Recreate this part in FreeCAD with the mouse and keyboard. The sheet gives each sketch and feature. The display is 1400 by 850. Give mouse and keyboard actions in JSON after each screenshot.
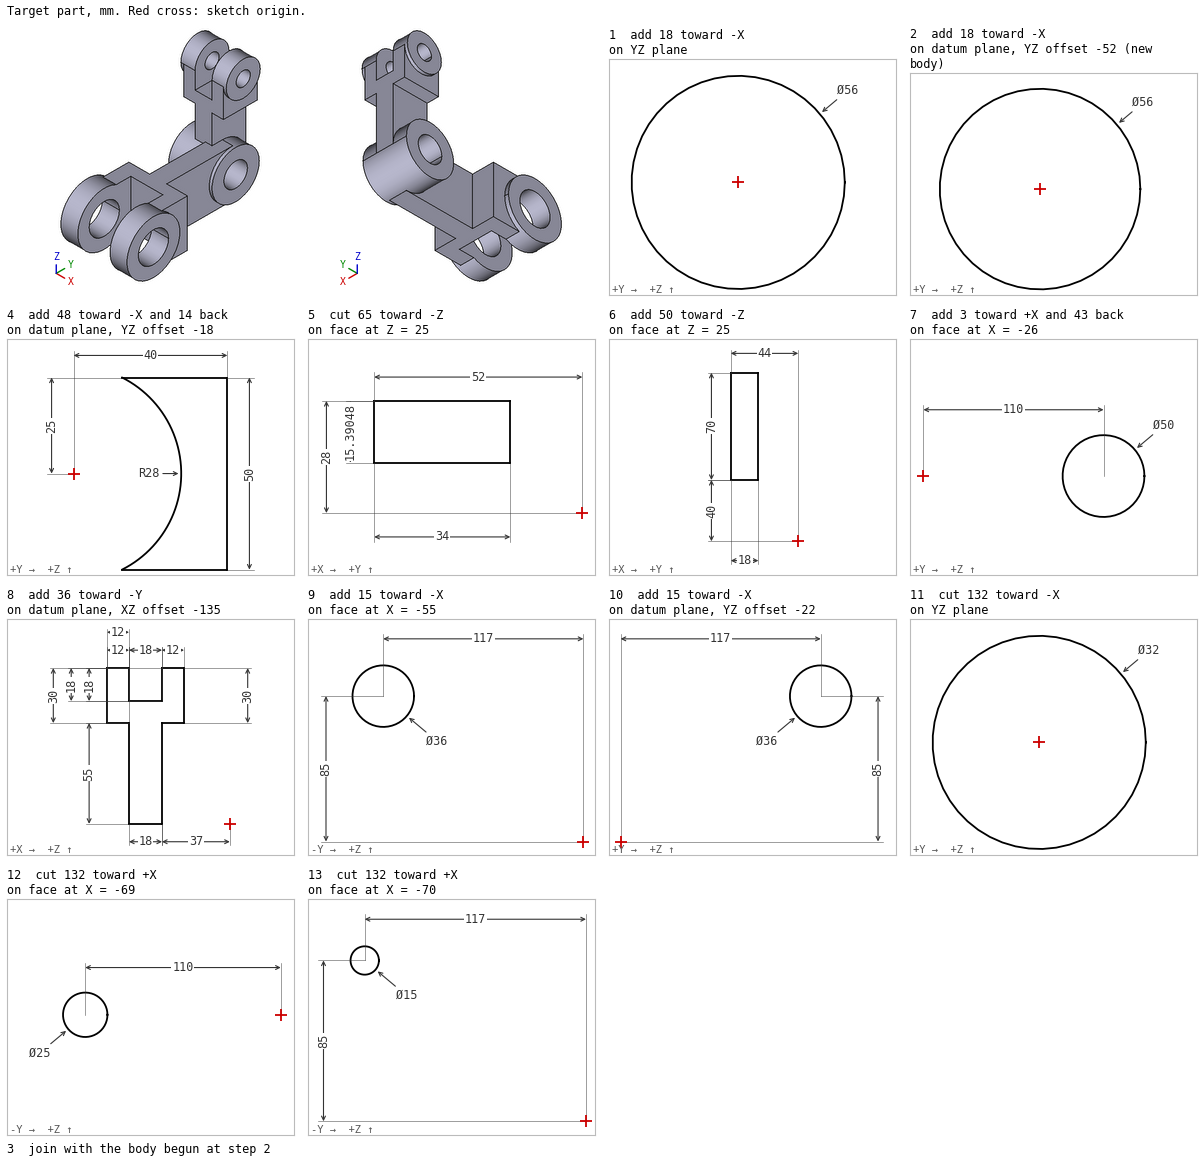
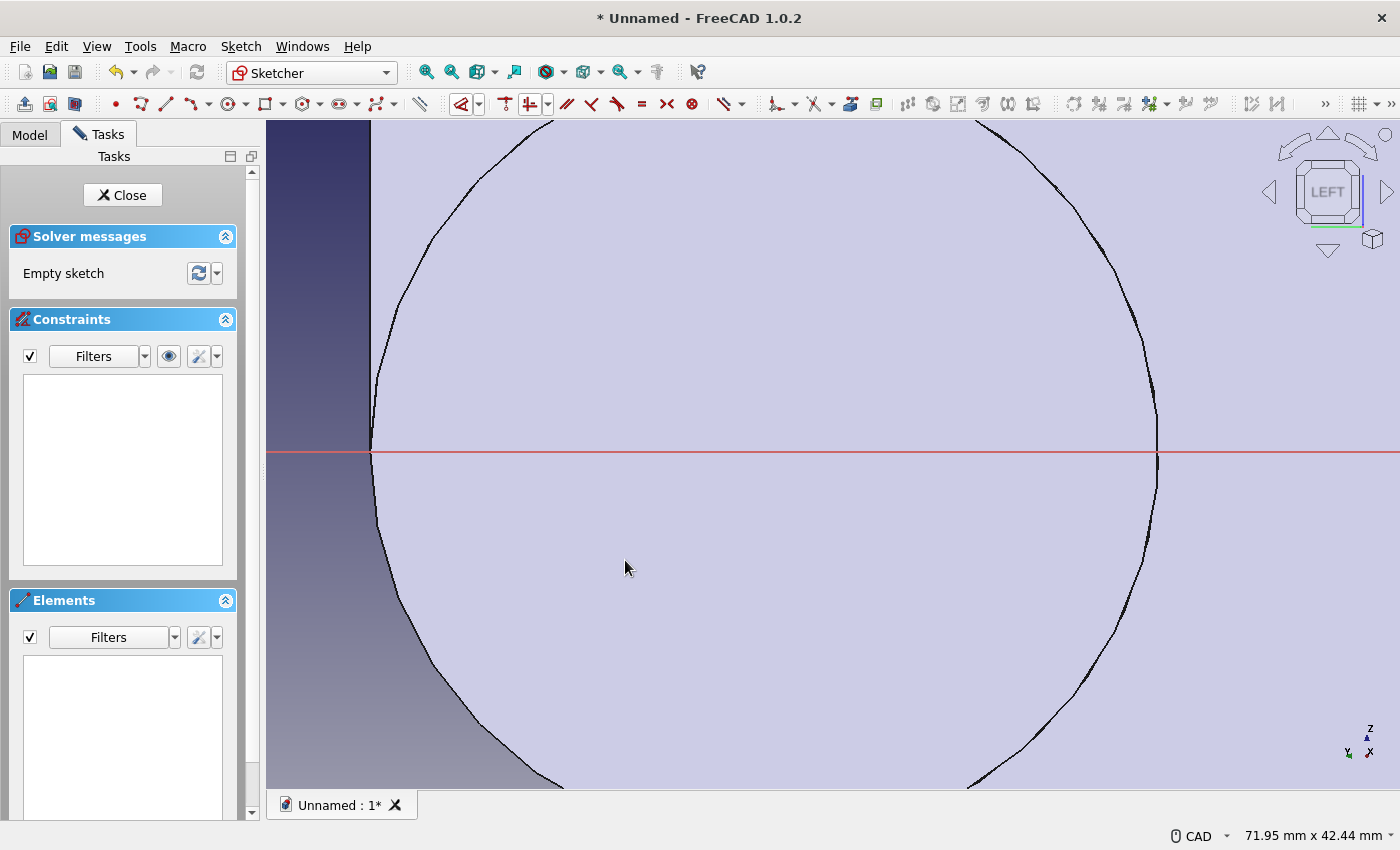
{"action": "left_click", "coordinate": [228, 104]}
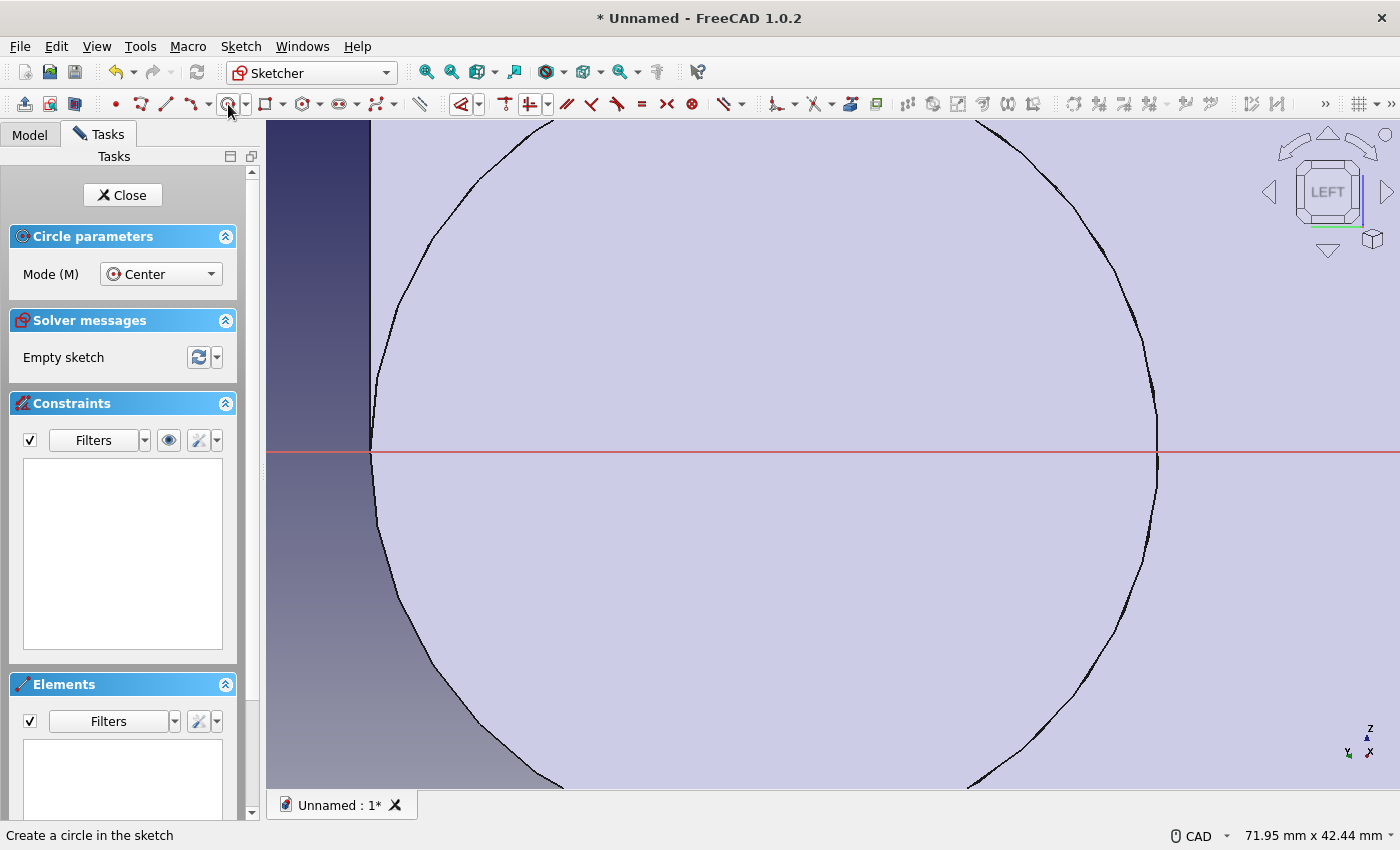
{"action": "left_click", "coordinate": [764, 452]}
{"action": "left_click", "coordinate": [904, 312]}
{"action": "key", "text": "Escape"}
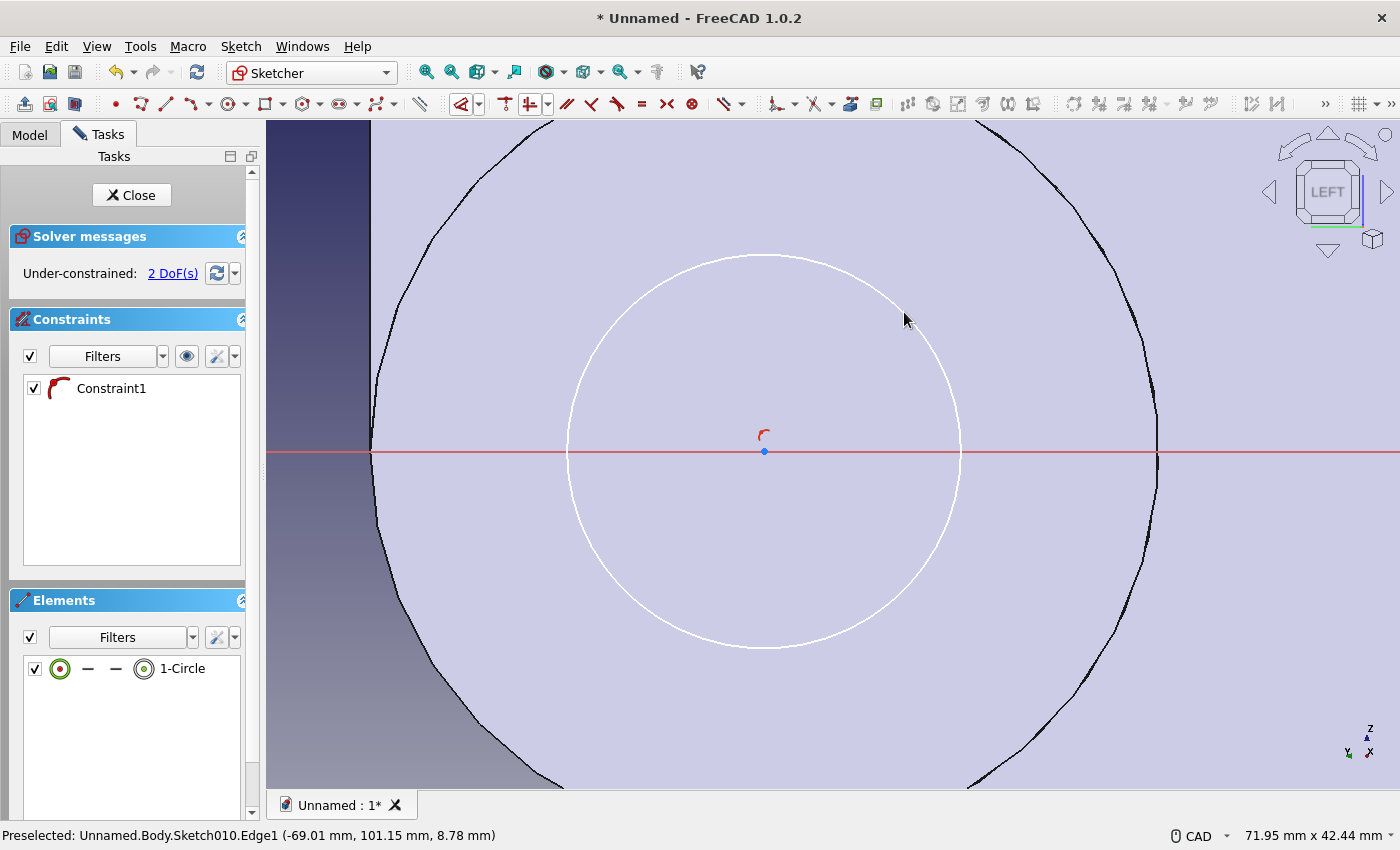
{"action": "left_click", "coordinate": [903, 312]}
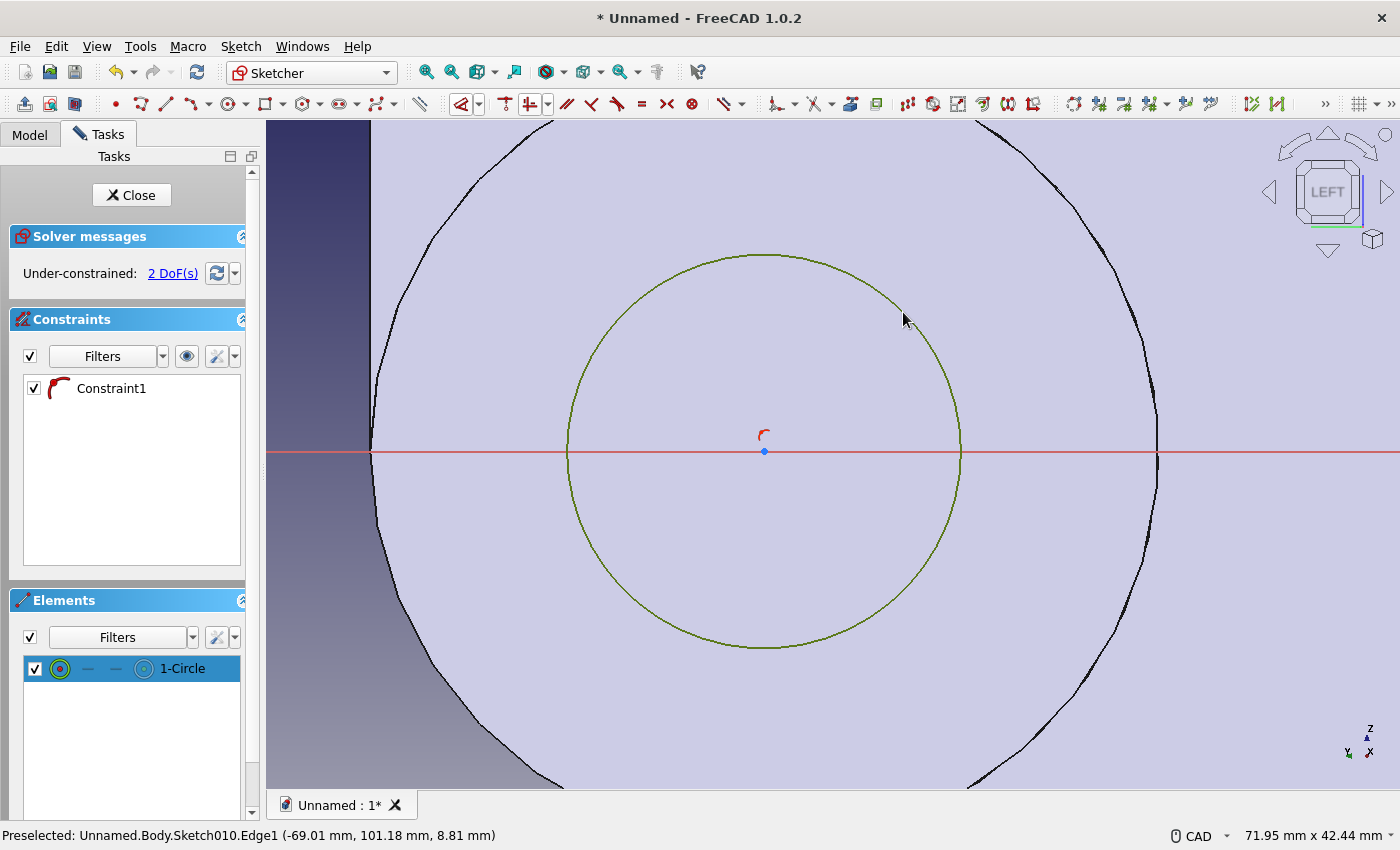
{"action": "key", "text": "k o"}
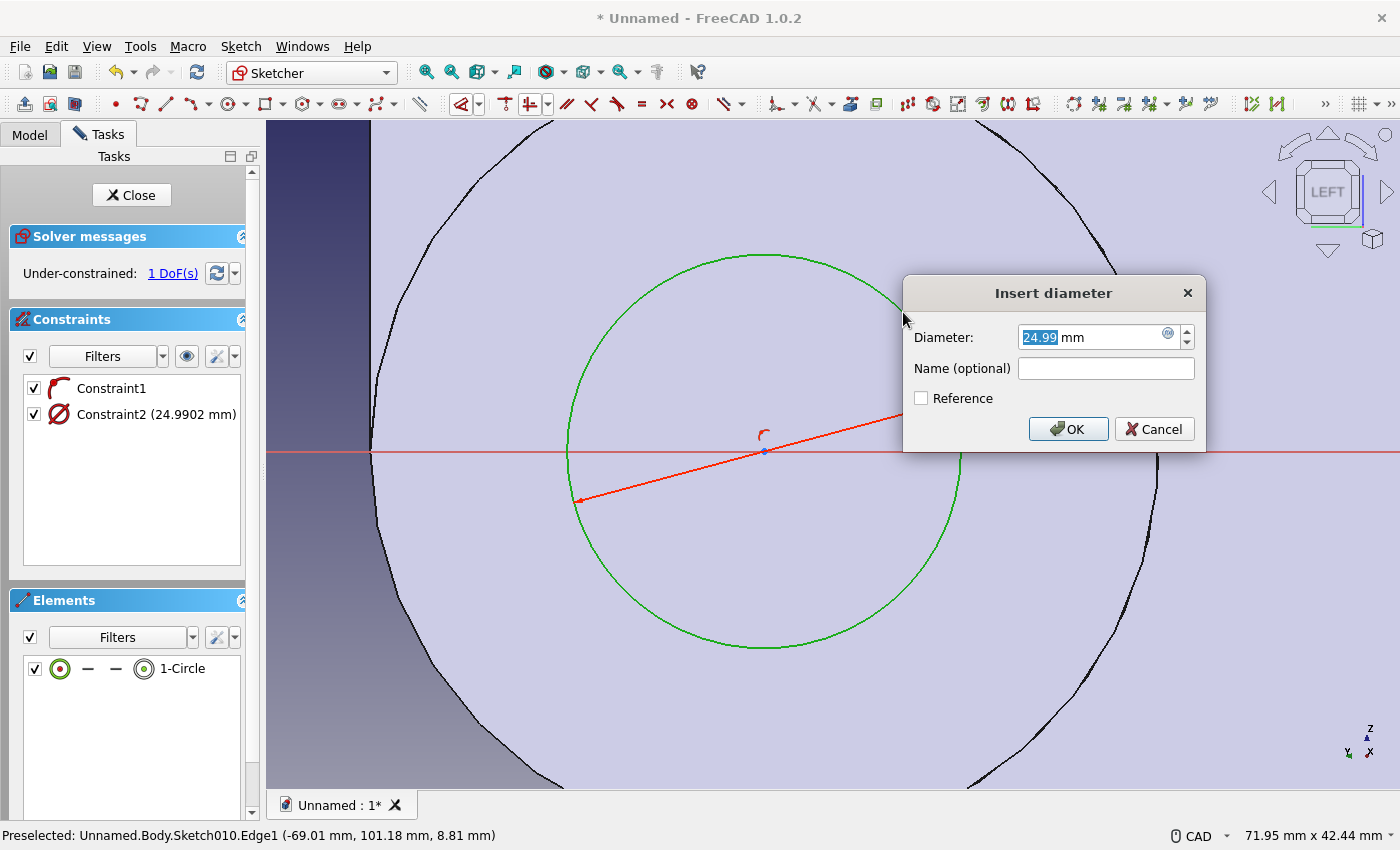
{"action": "type", "text": "25"}
{"action": "key", "text": "Return"}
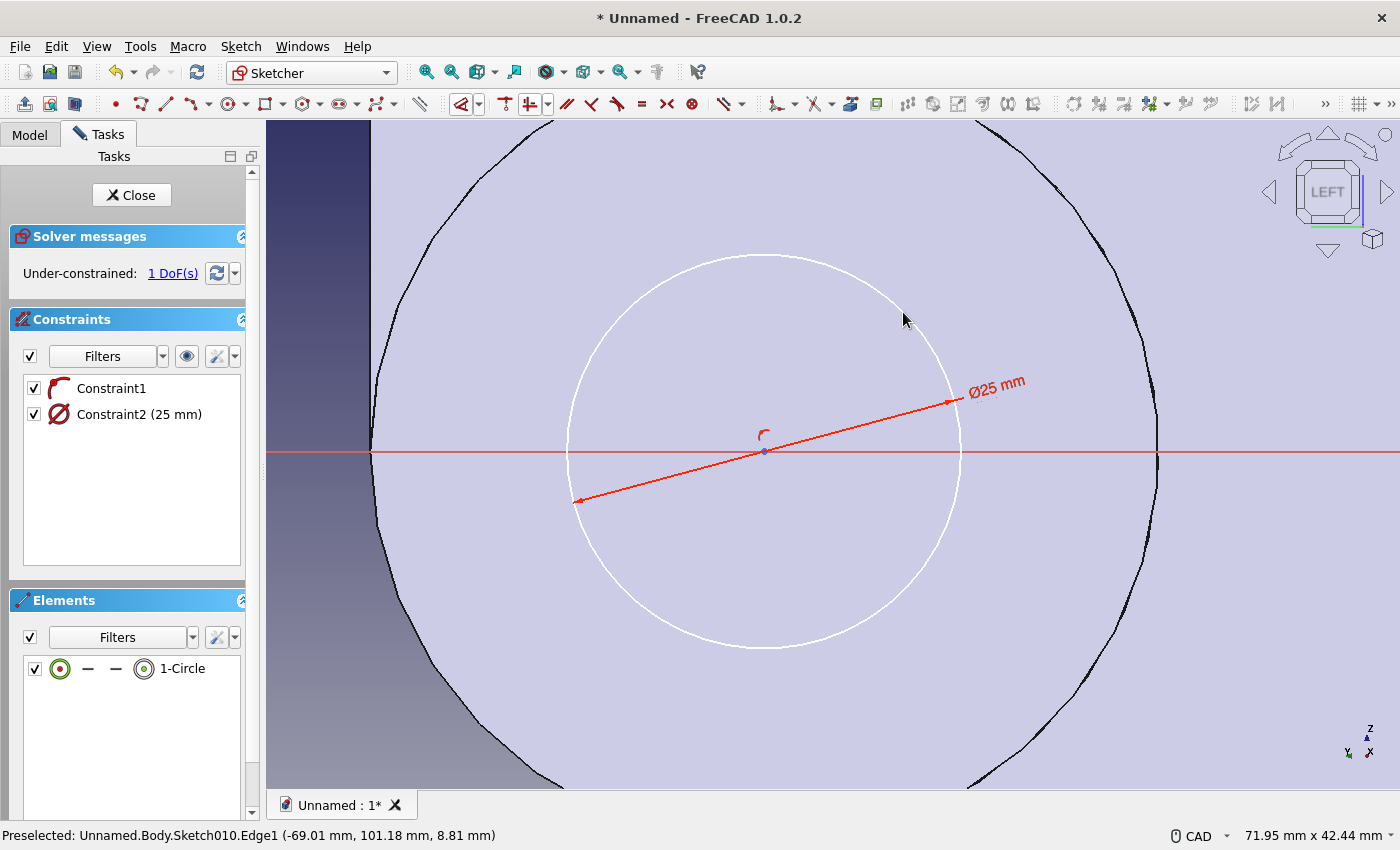
{"action": "left_click", "coordinate": [764, 452]}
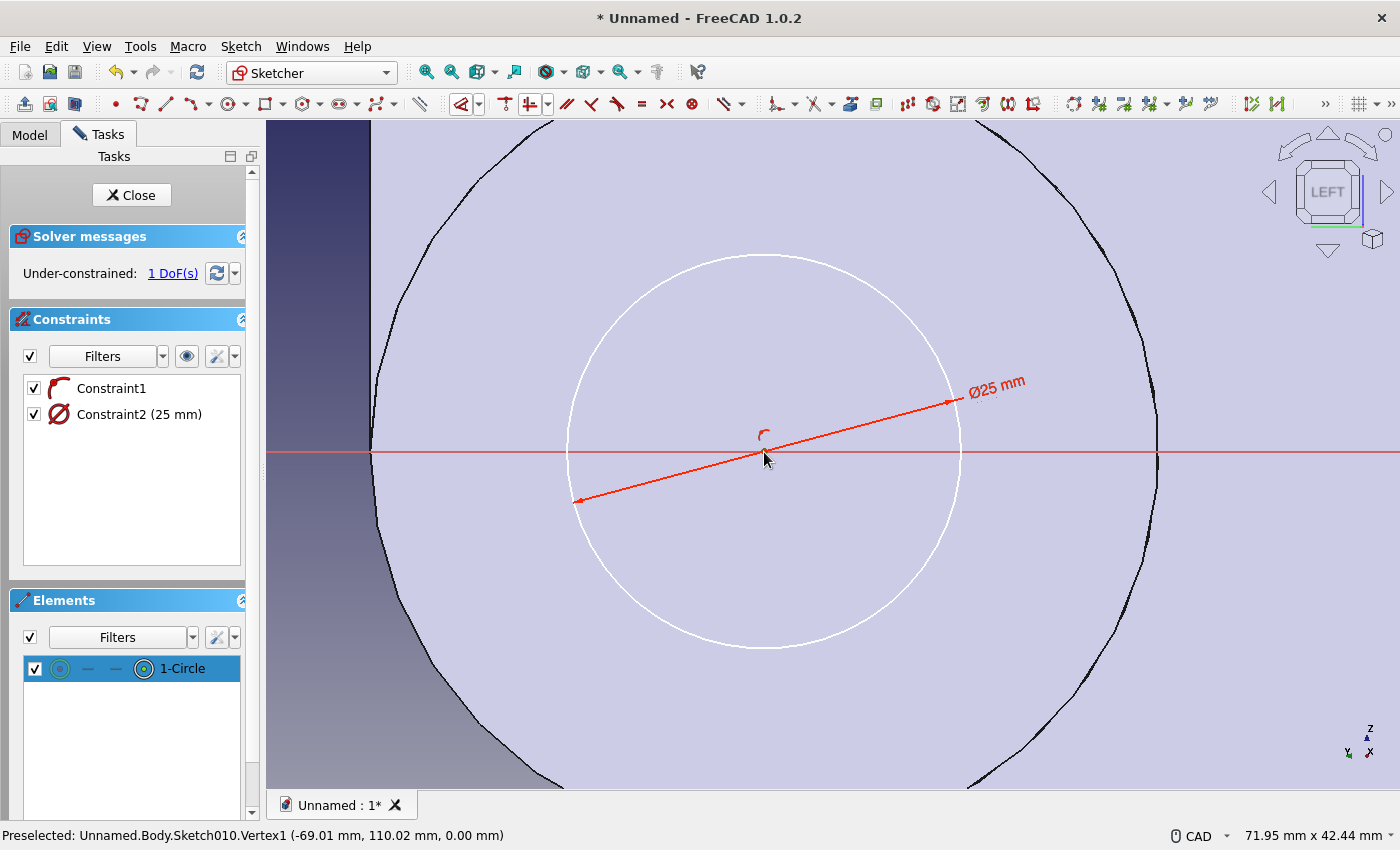
{"action": "key", "text": "l"}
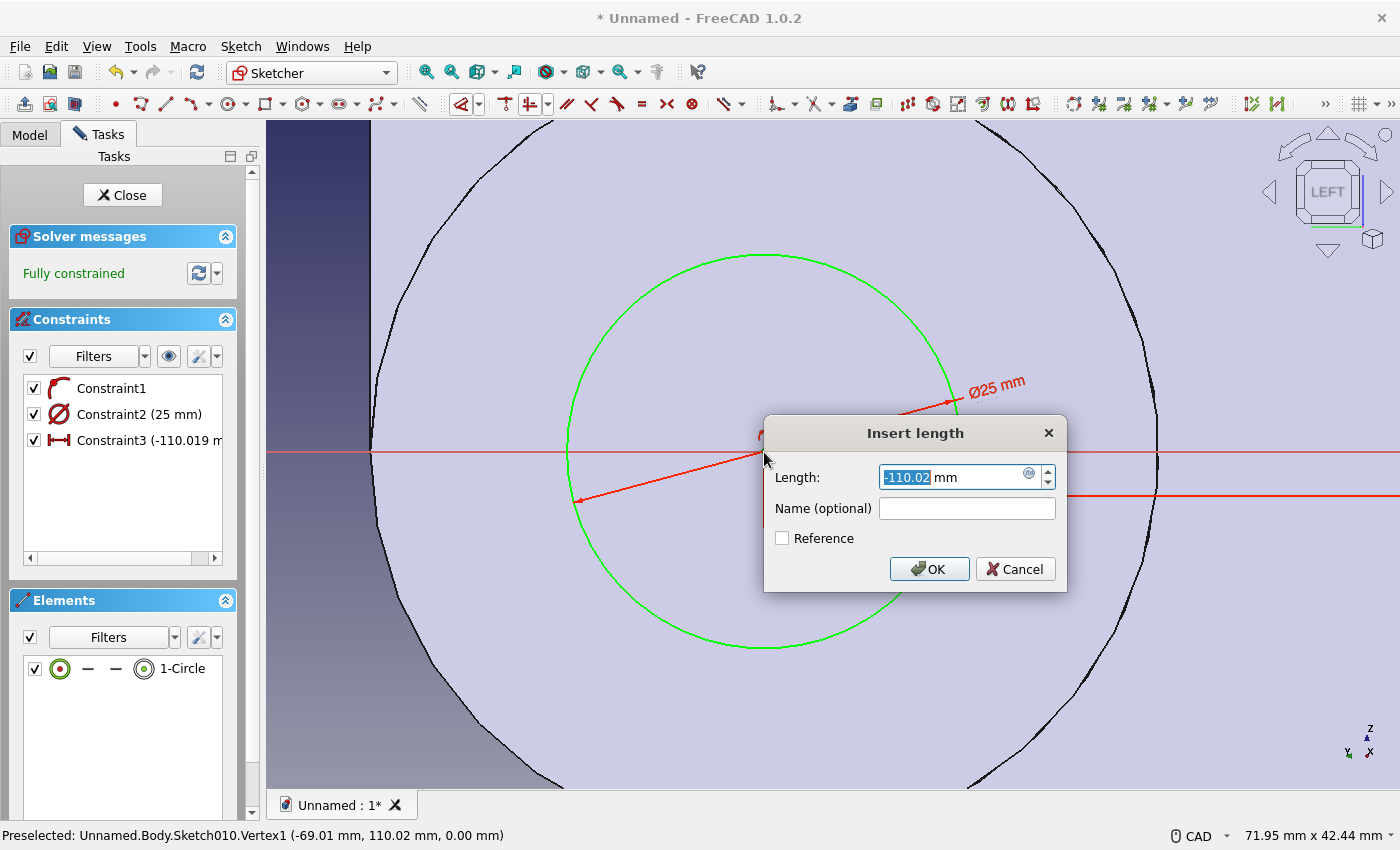
{"action": "type", "text": "-110"}
{"action": "key", "text": "Return"}